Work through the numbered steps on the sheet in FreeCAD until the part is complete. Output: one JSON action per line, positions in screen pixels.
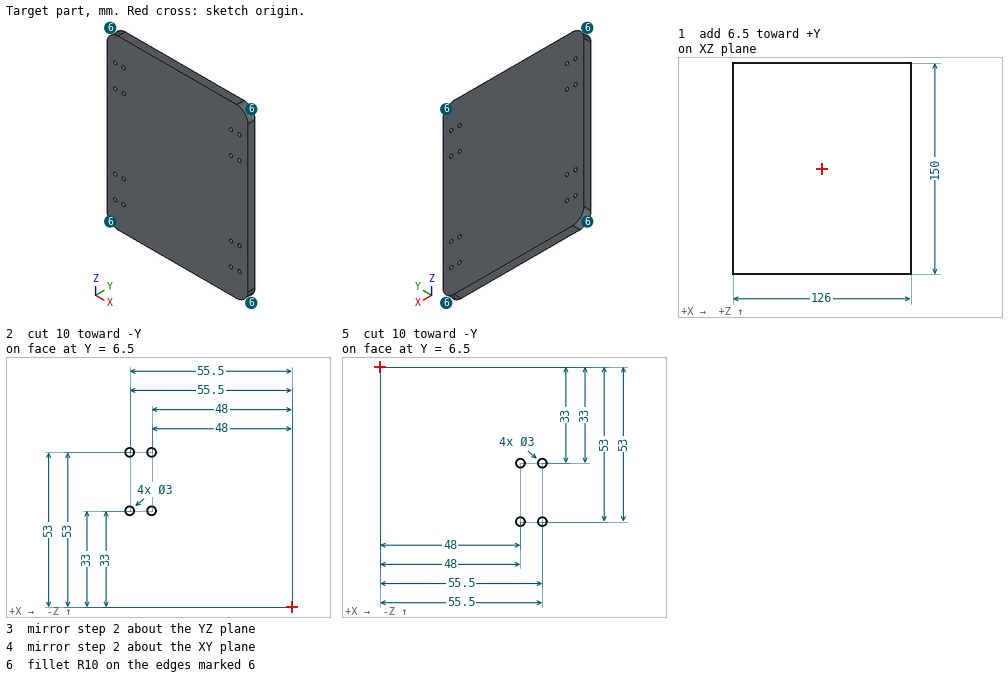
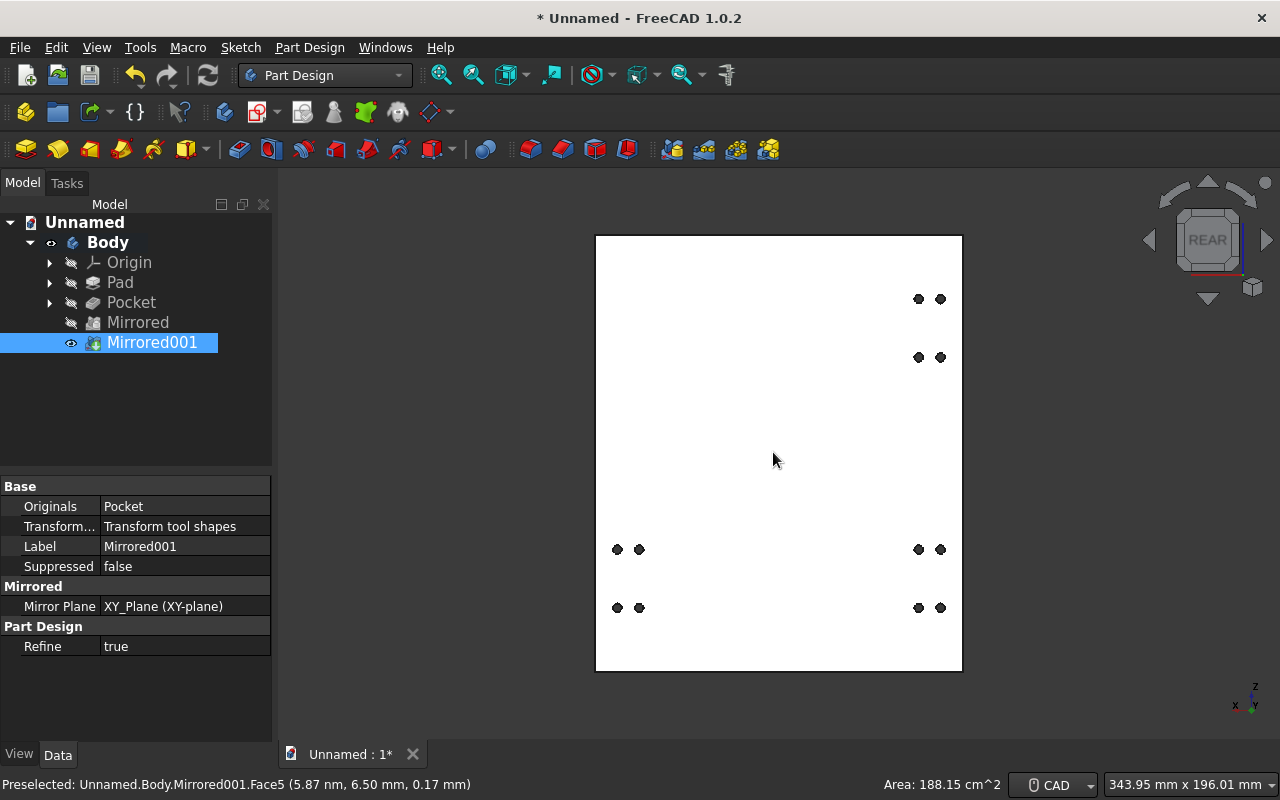
{"action": "left_click", "coordinate": [258, 112]}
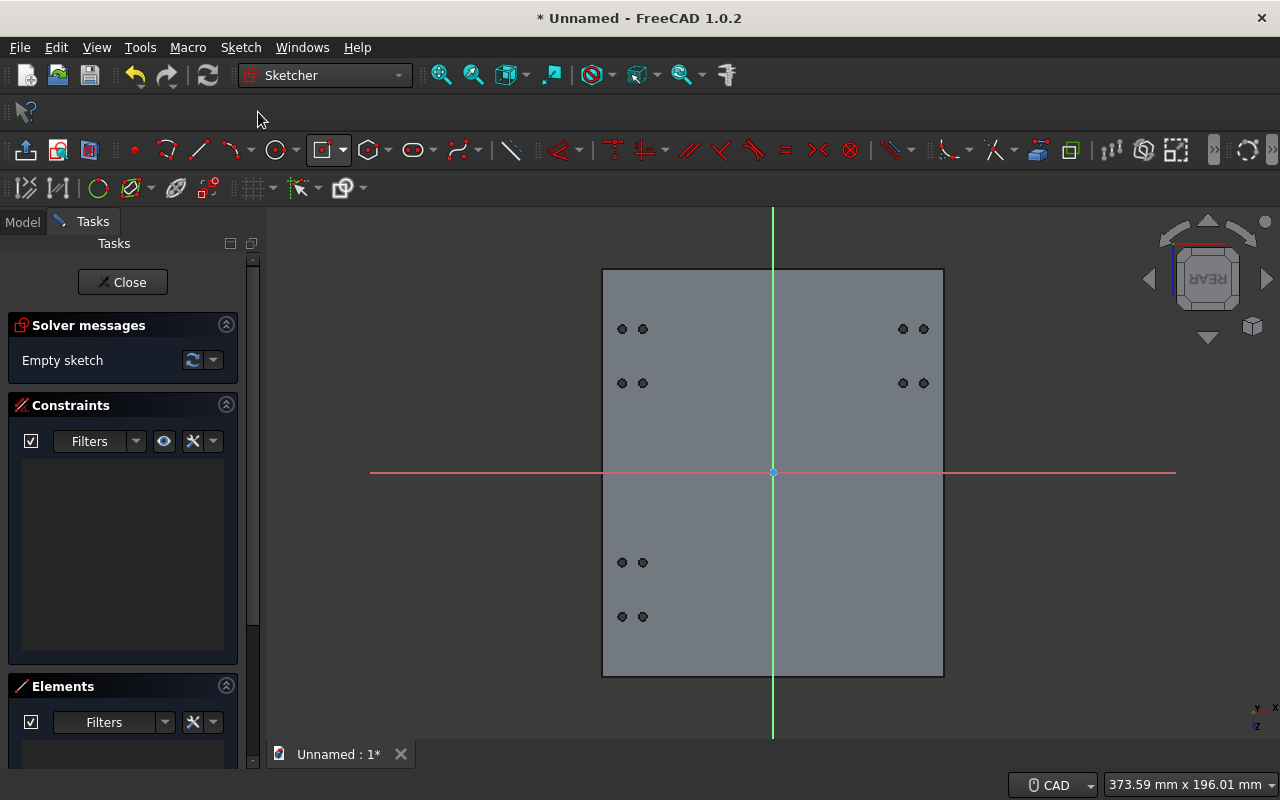
{"action": "scroll", "coordinate": [969, 607], "scroll_direction": "up", "scroll_amount": 4}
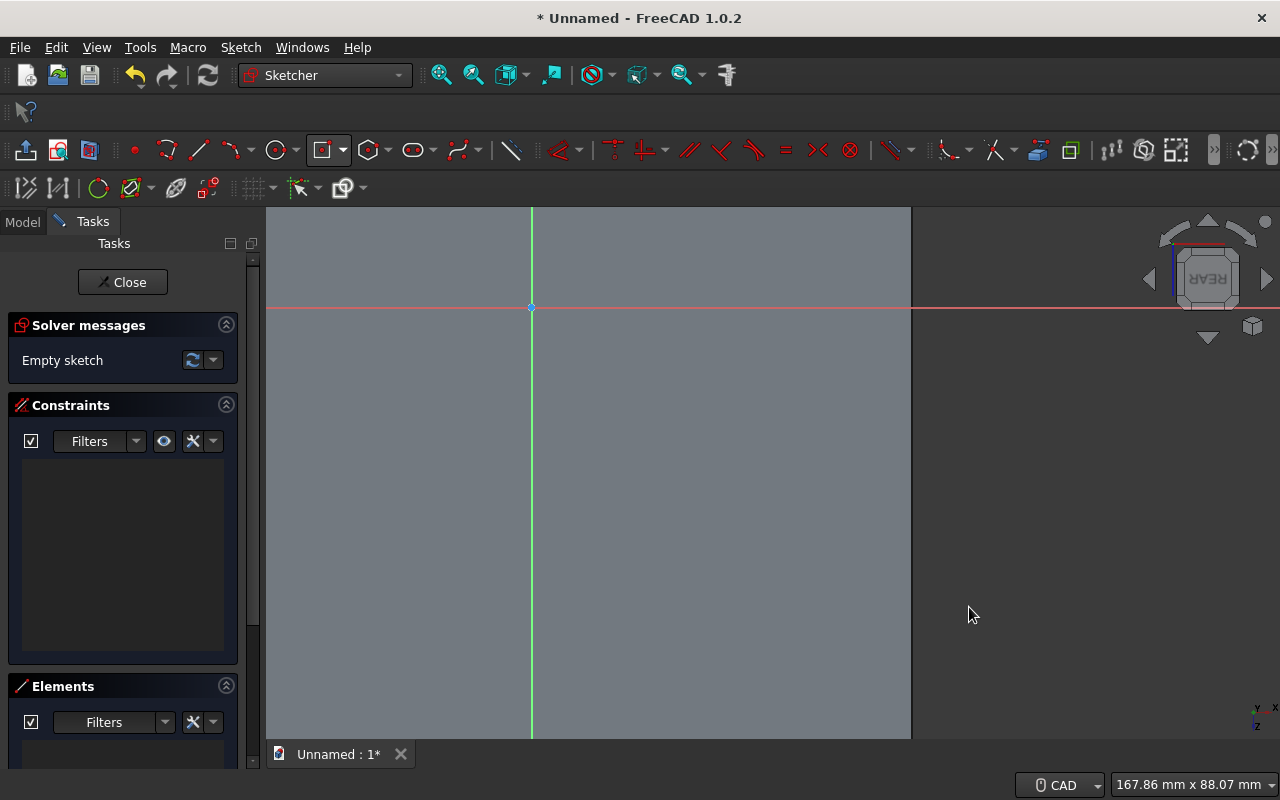
{"action": "left_click", "coordinate": [276, 150]}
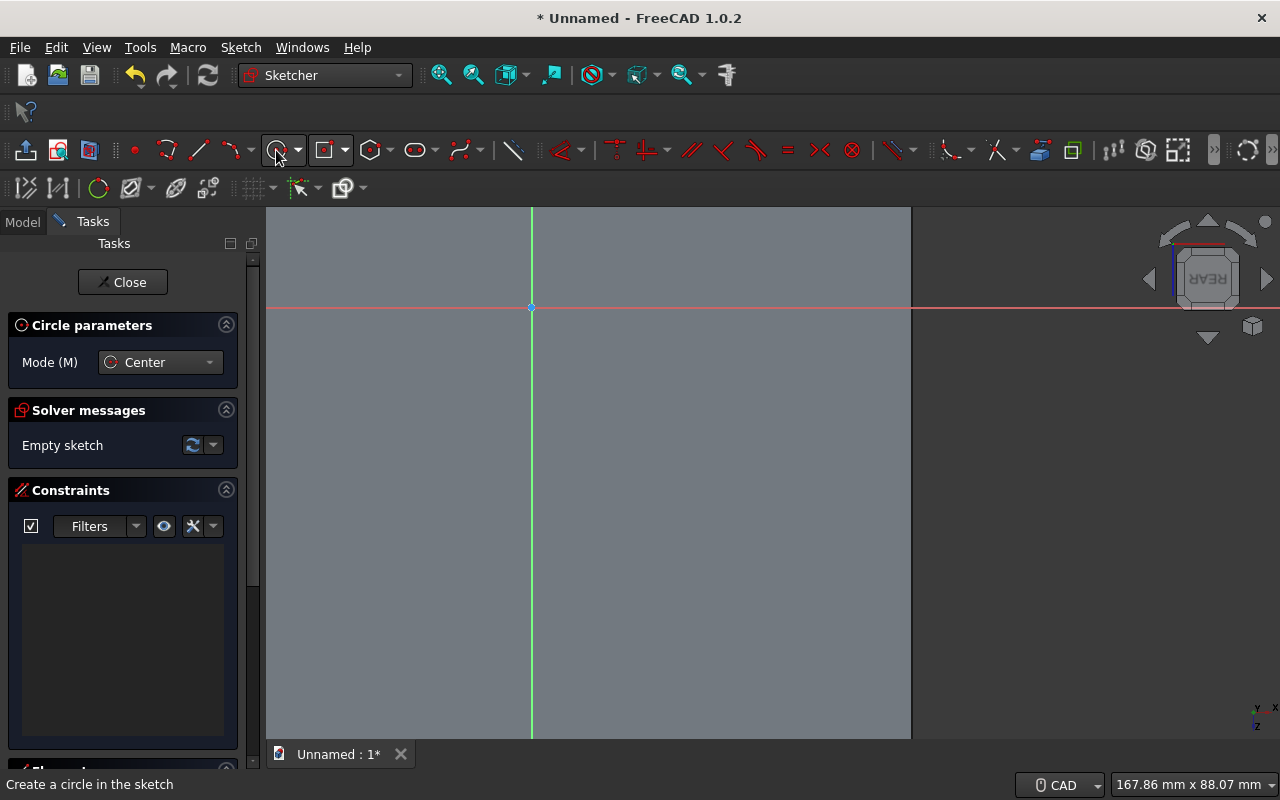
{"action": "scroll", "coordinate": [867, 507], "scroll_direction": "up", "scroll_amount": 5}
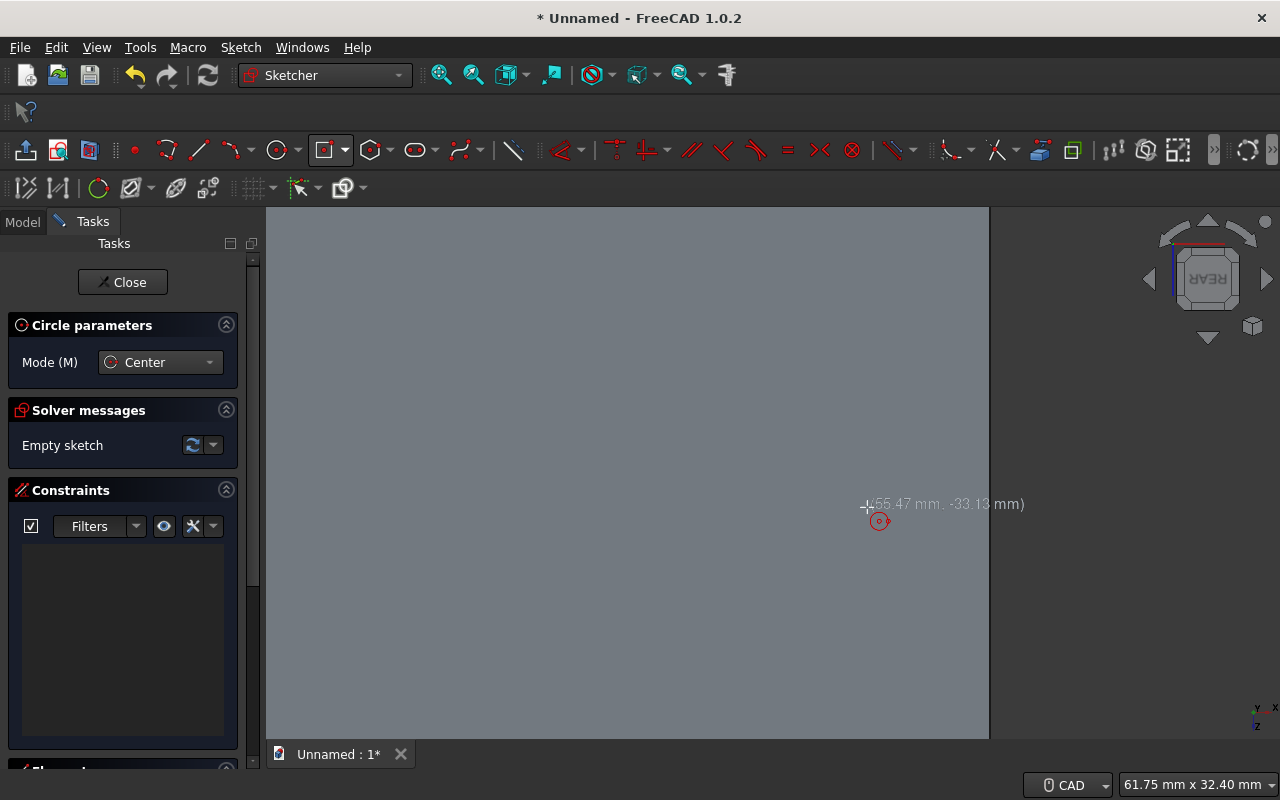
{"action": "left_click", "coordinate": [867, 507]}
{"action": "left_click", "coordinate": [884, 489]}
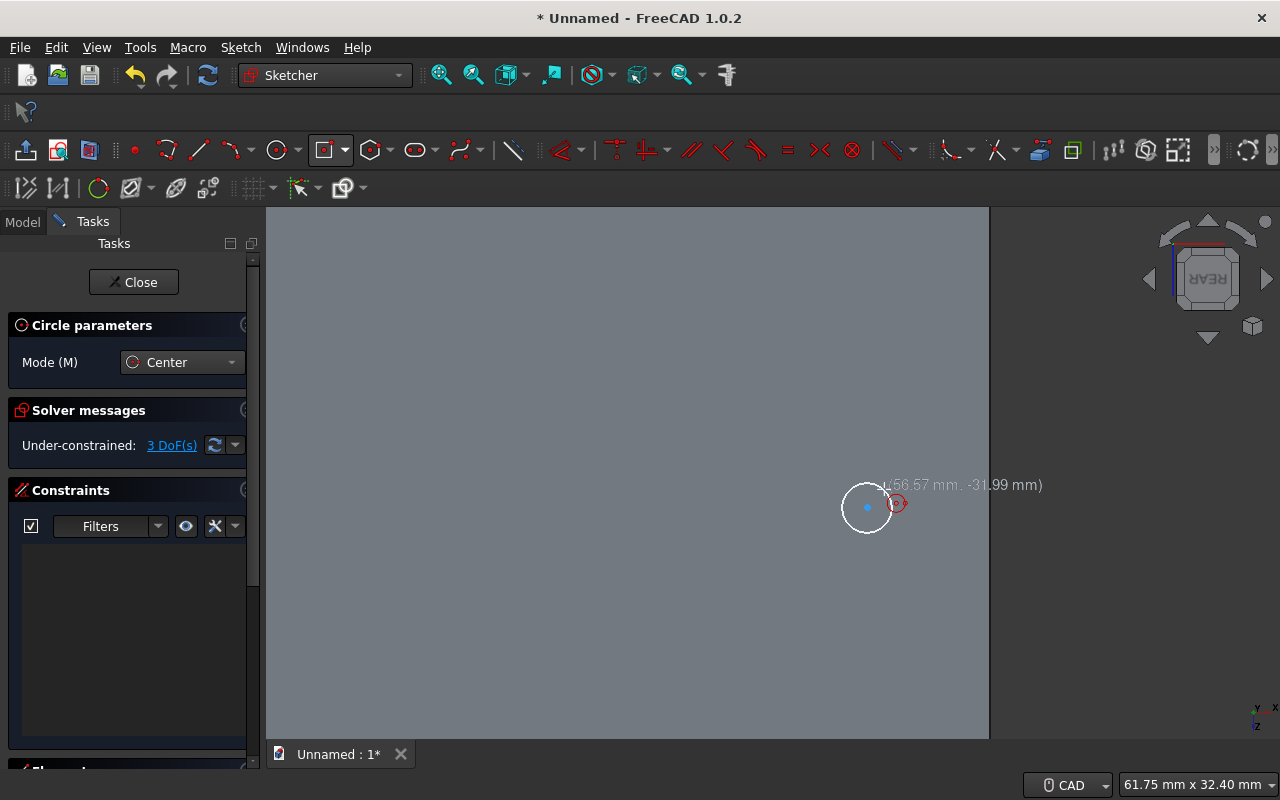
{"action": "left_click", "coordinate": [743, 507]}
{"action": "left_click", "coordinate": [761, 489]}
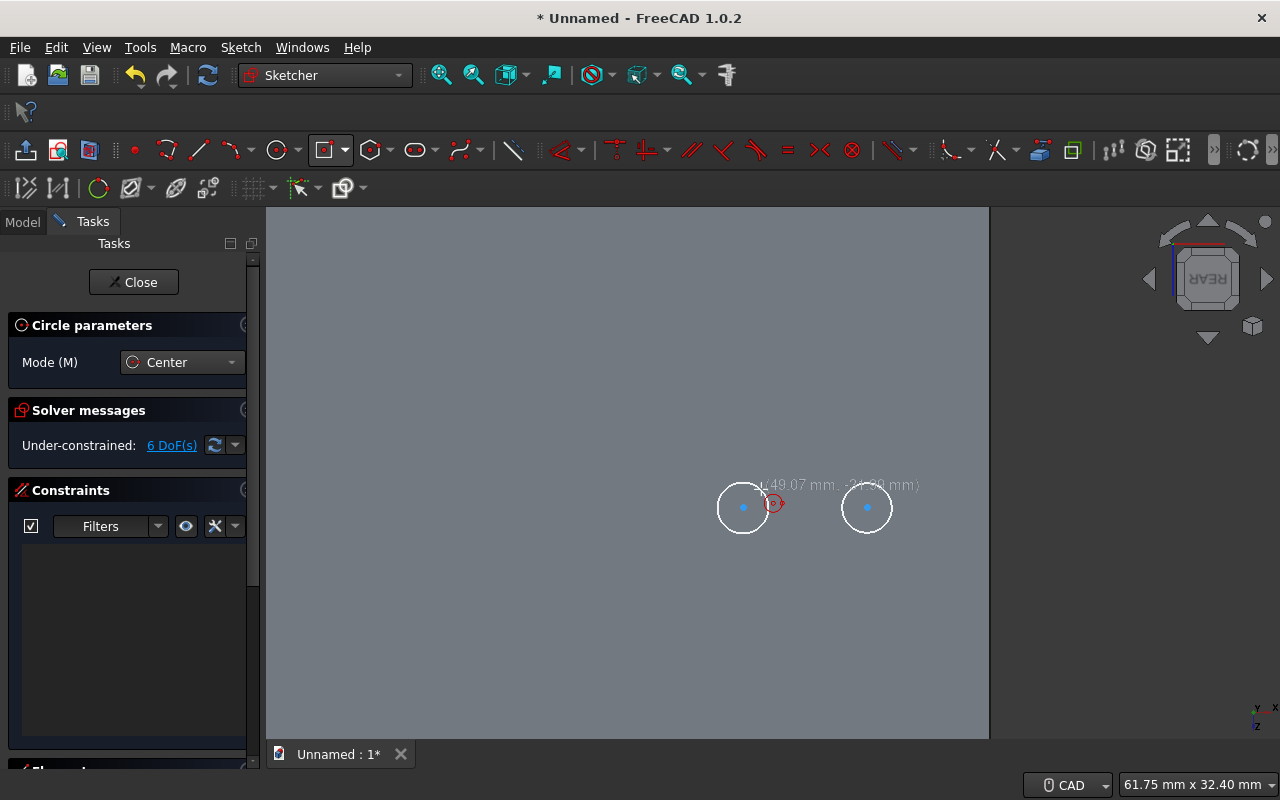
{"action": "scroll", "coordinate": [868, 508], "scroll_direction": "down", "scroll_amount": 5}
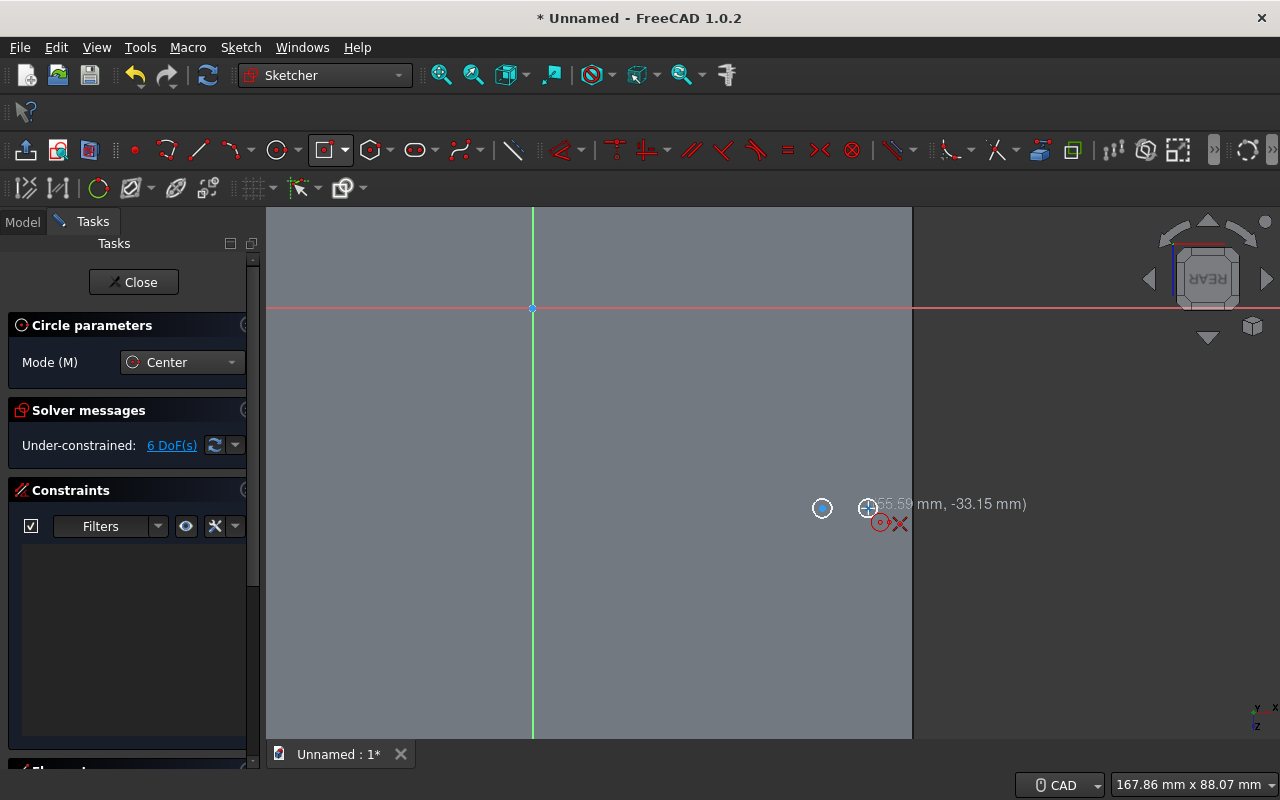
{"action": "scroll", "coordinate": [823, 629], "scroll_direction": "up", "scroll_amount": 5}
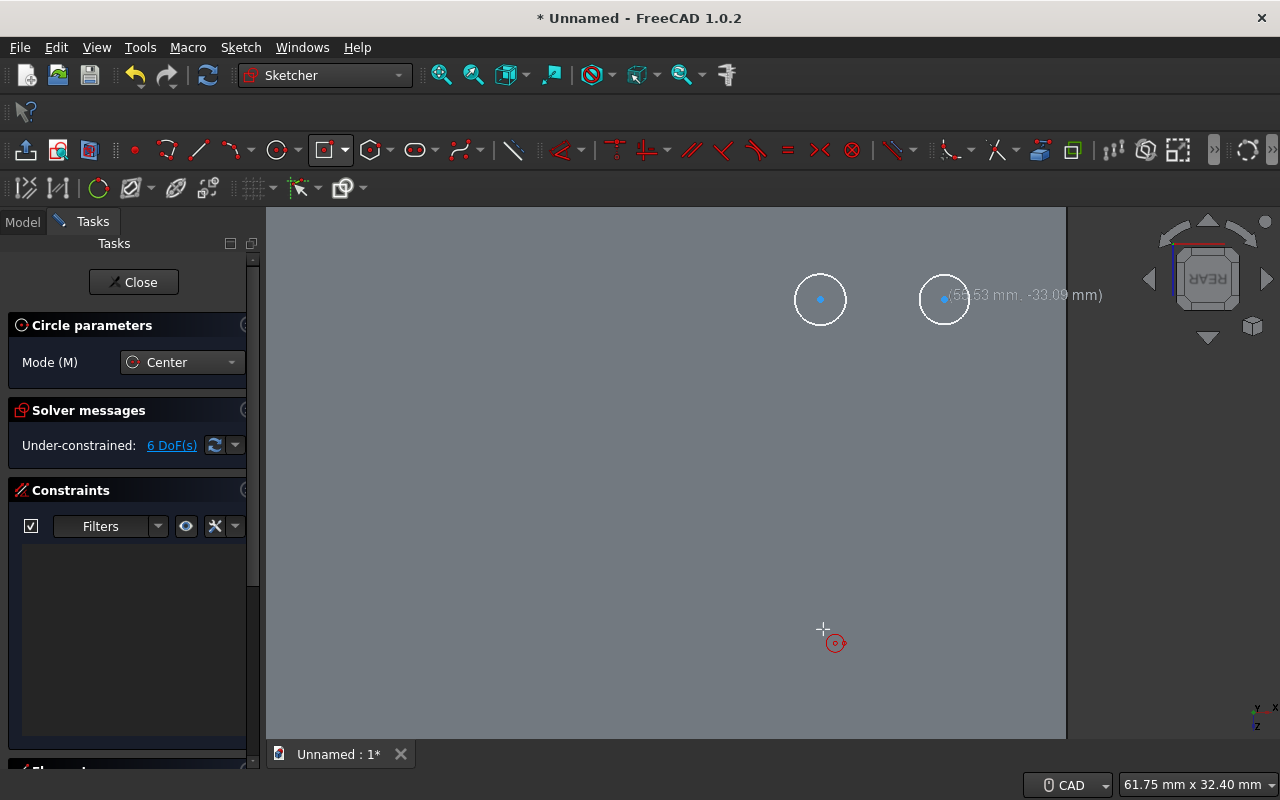
{"action": "left_click", "coordinate": [821, 627]}
{"action": "left_click", "coordinate": [838, 609]}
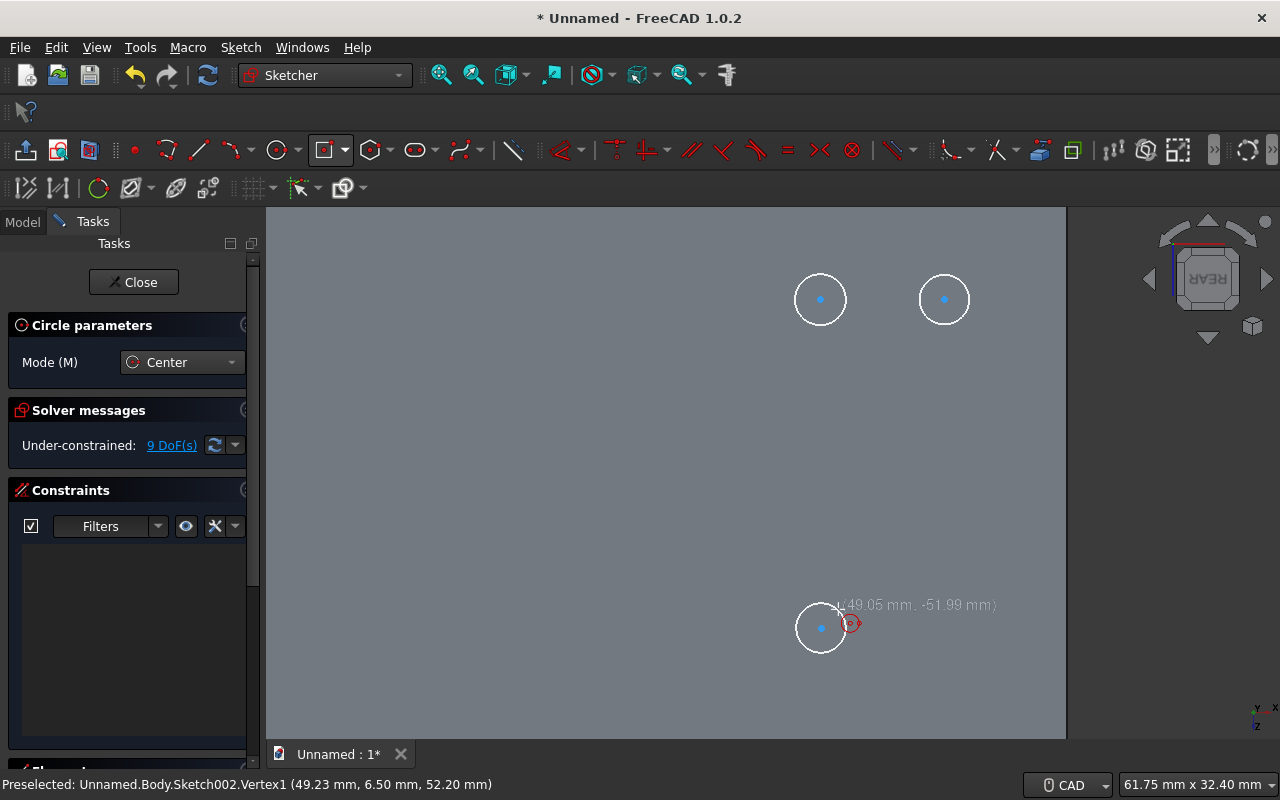
{"action": "left_click", "coordinate": [944, 627]}
{"action": "left_click", "coordinate": [961, 609]}
{"action": "key", "text": "Escape"}